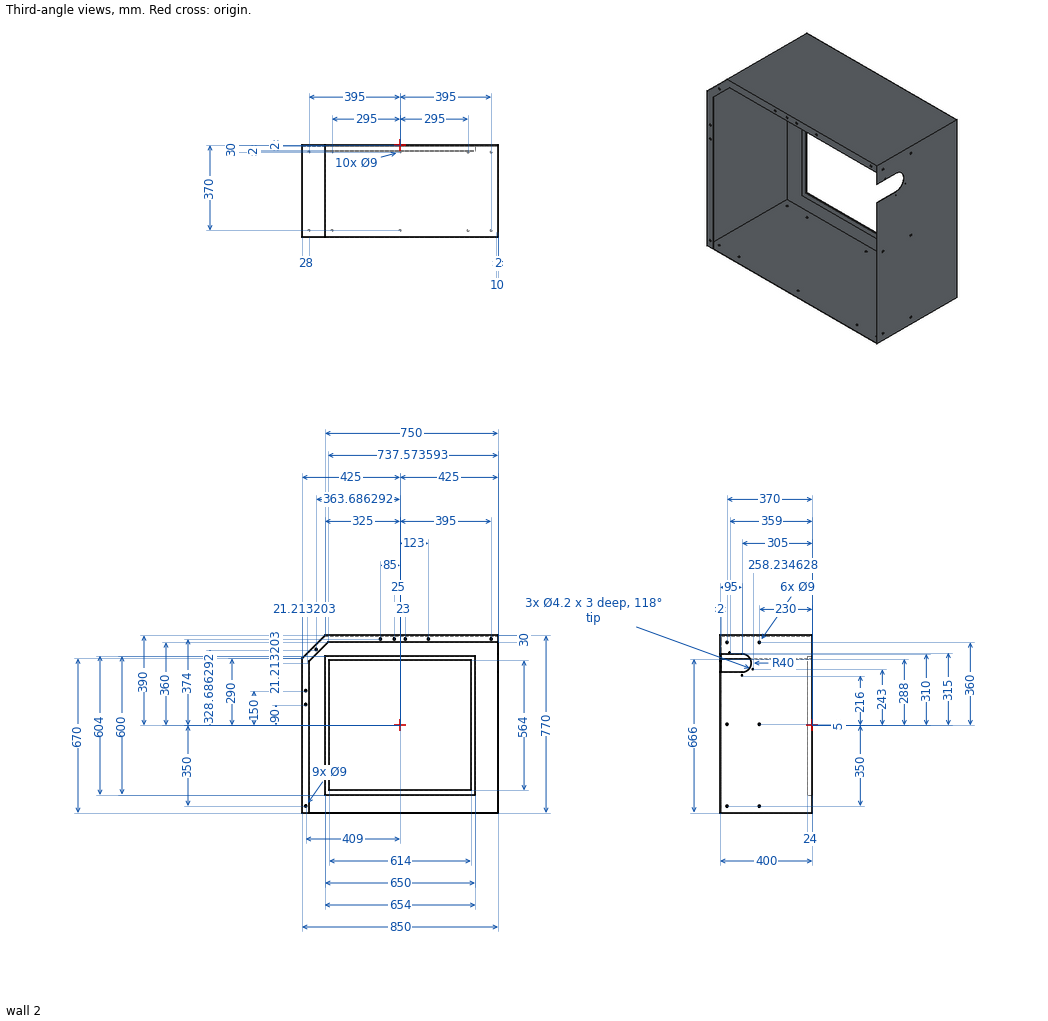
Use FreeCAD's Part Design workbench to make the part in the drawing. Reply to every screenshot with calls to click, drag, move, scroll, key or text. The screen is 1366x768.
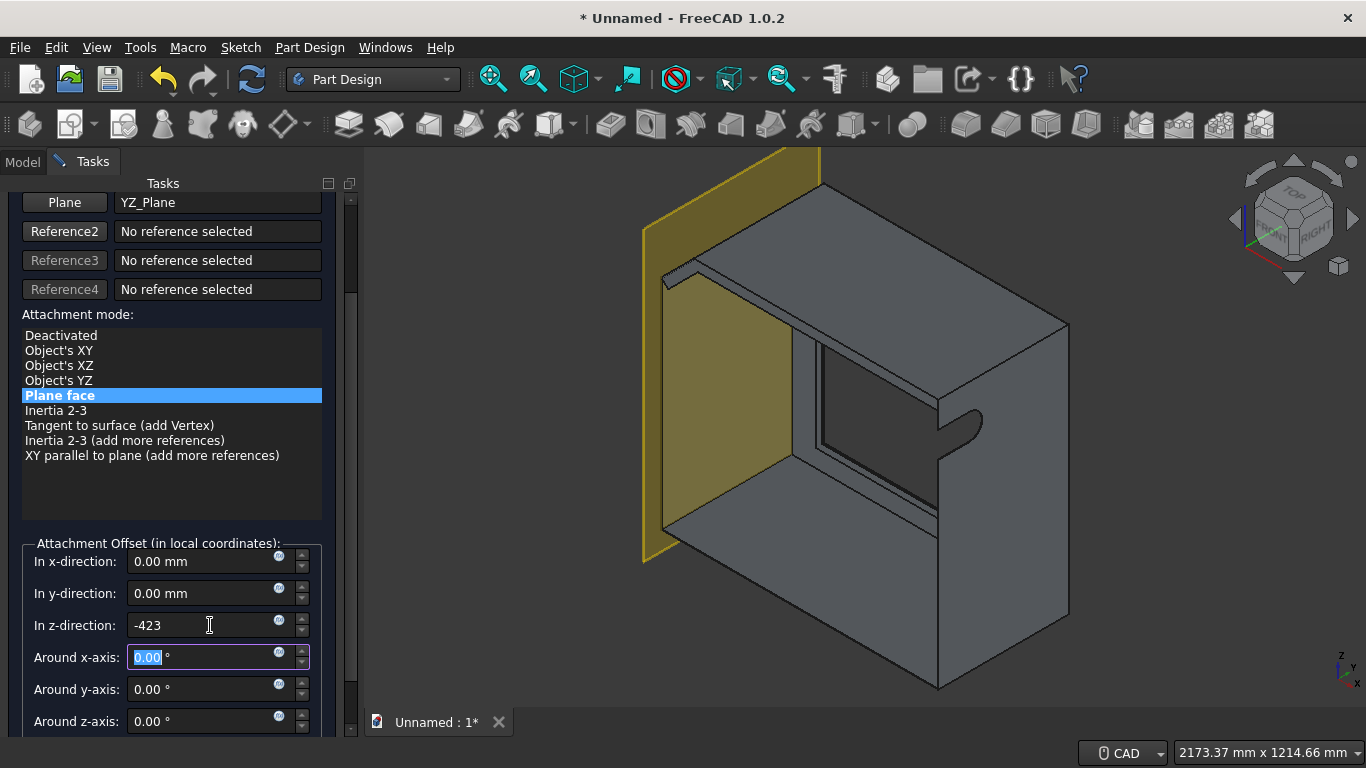
scroll(351, 464, up, 3)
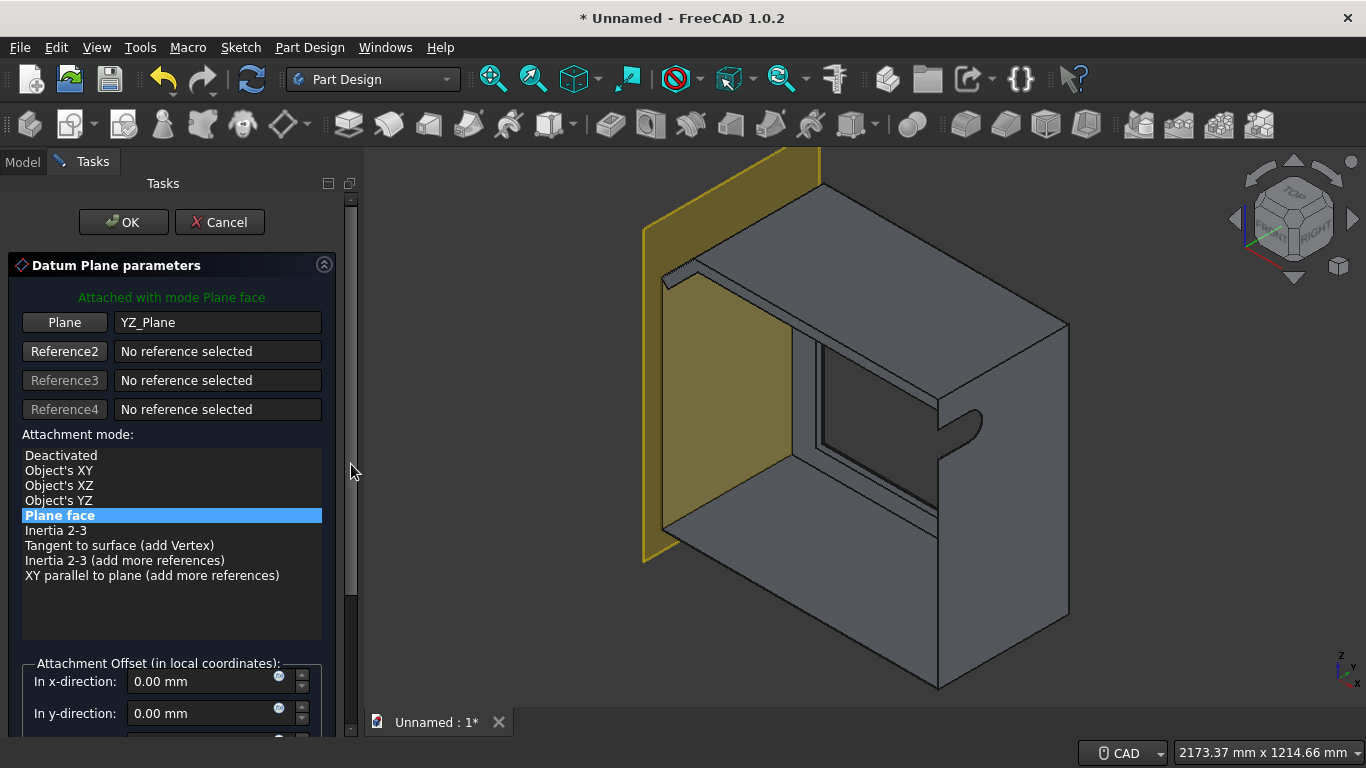
click(124, 222)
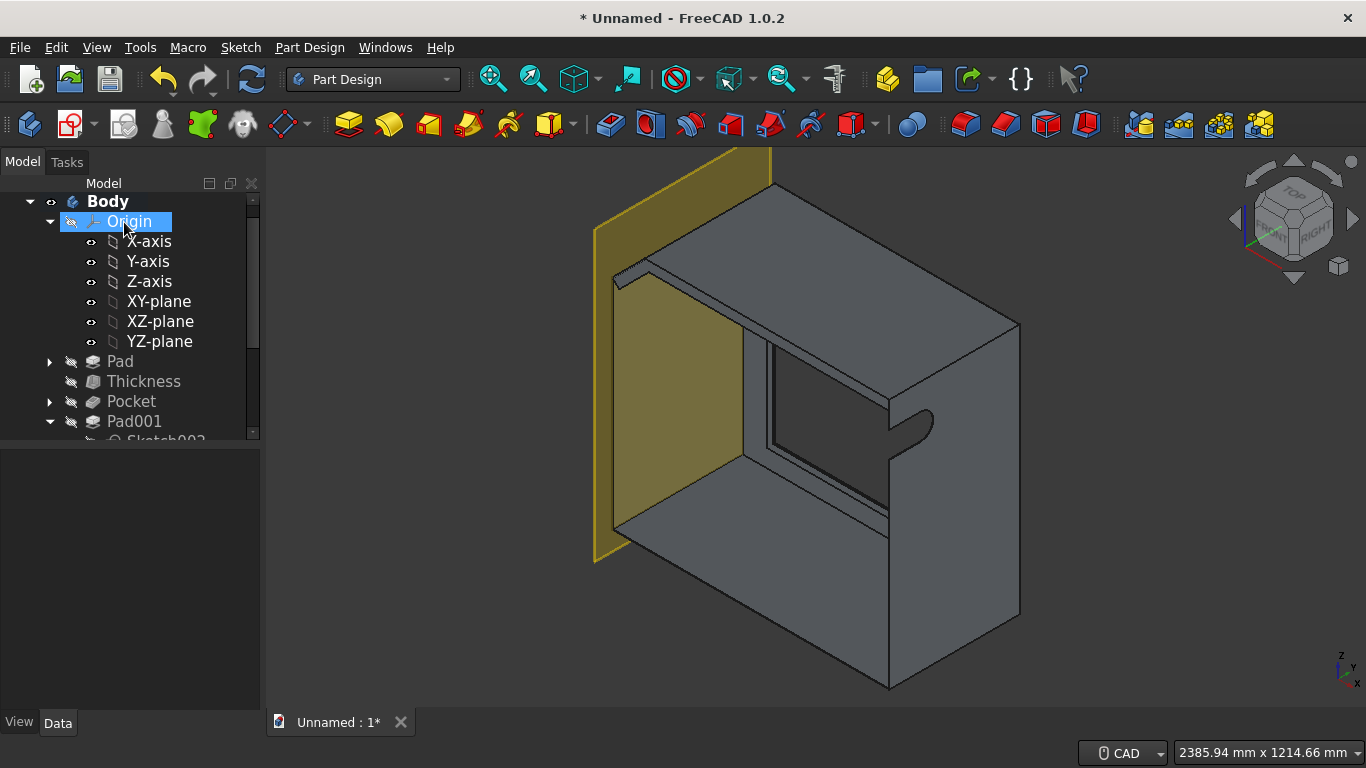
scroll(120, 317, down, 3)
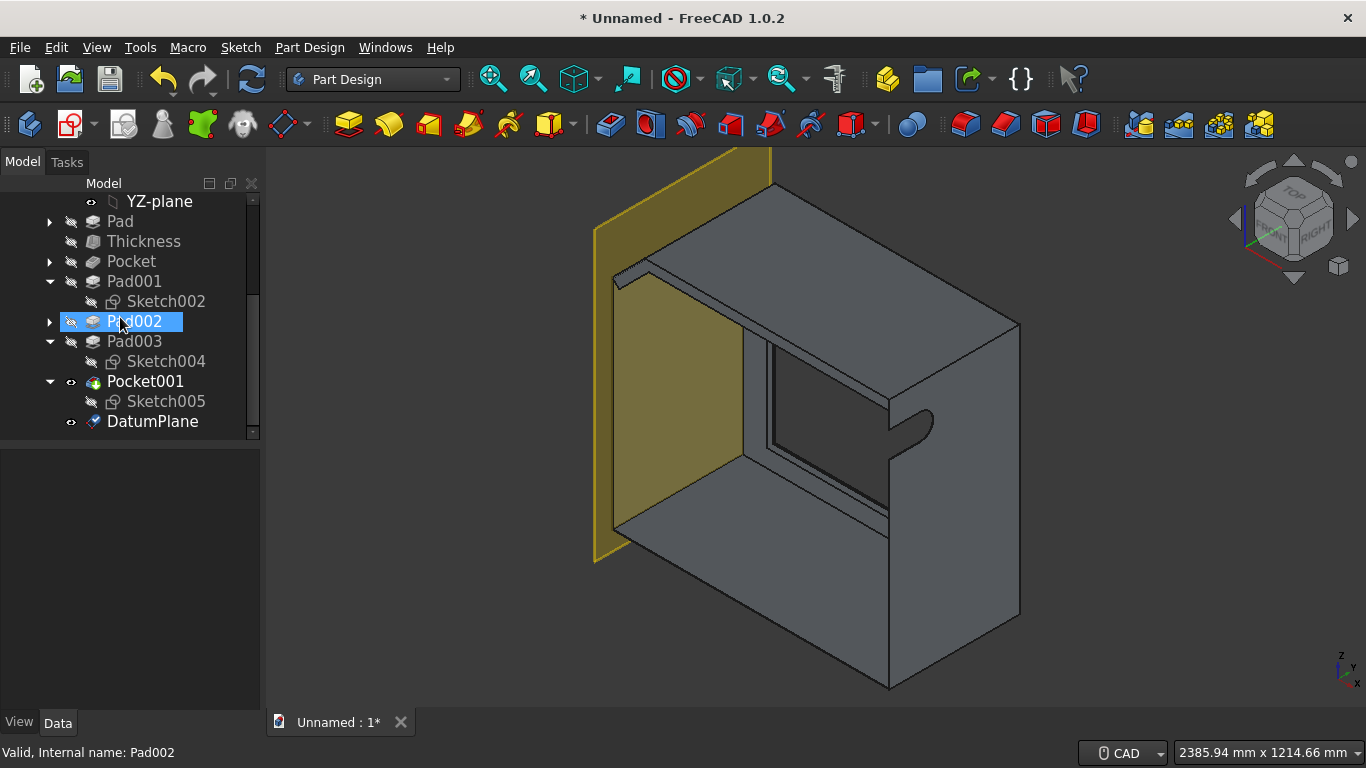
click(116, 422)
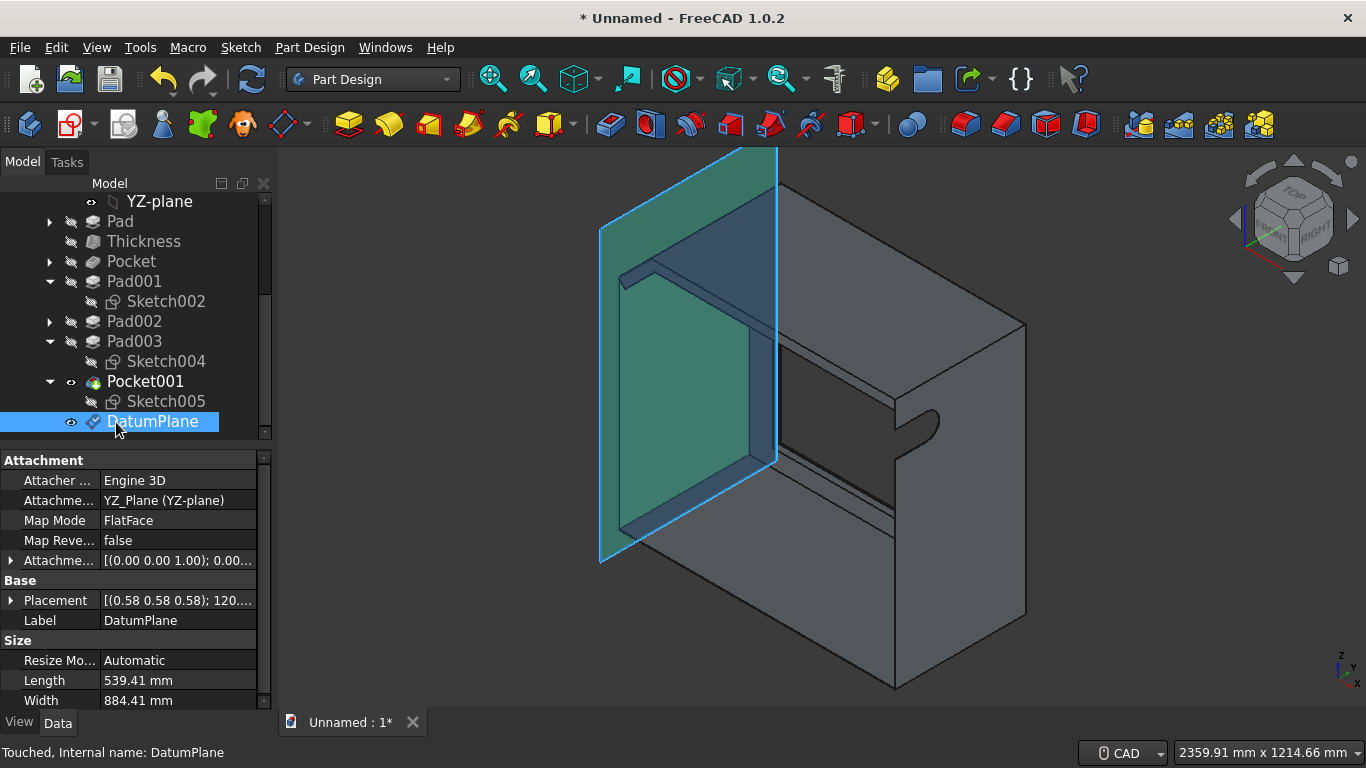
click(70, 124)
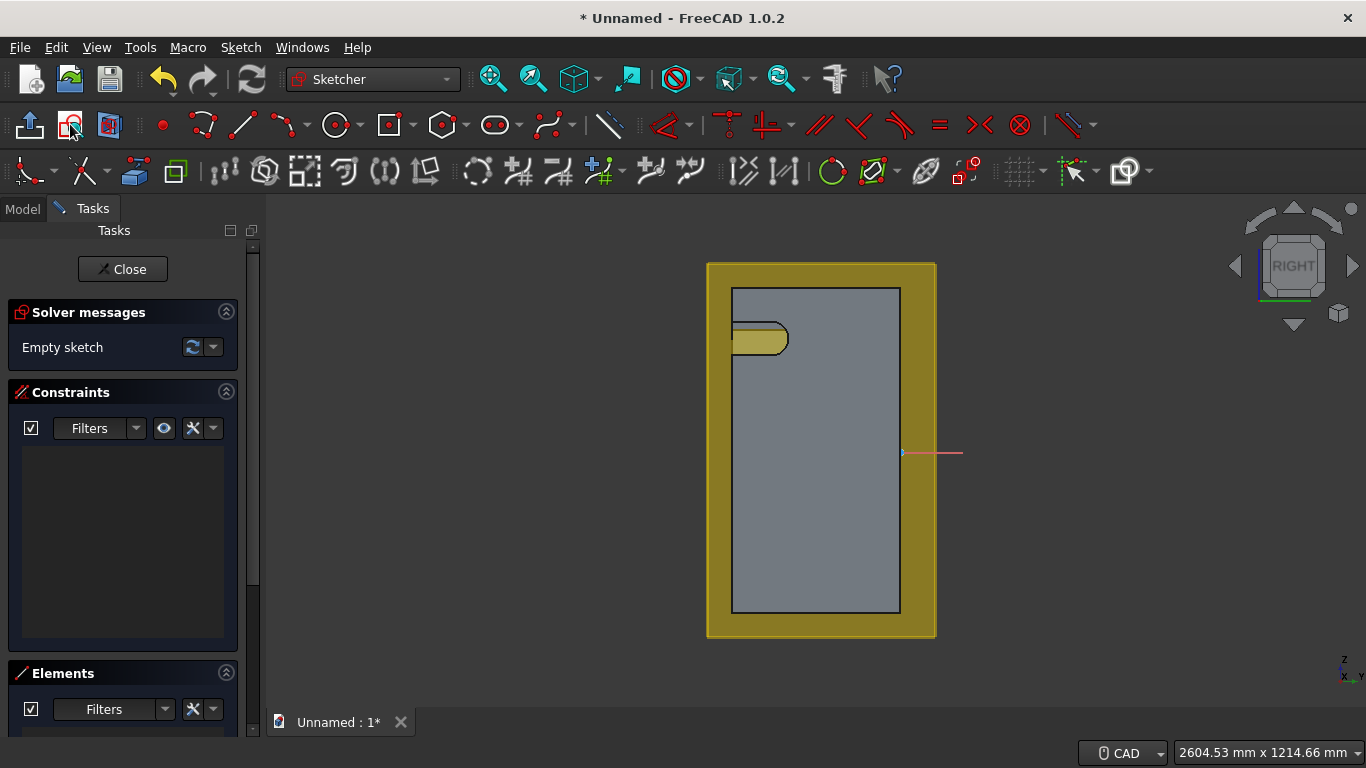
click(110, 126)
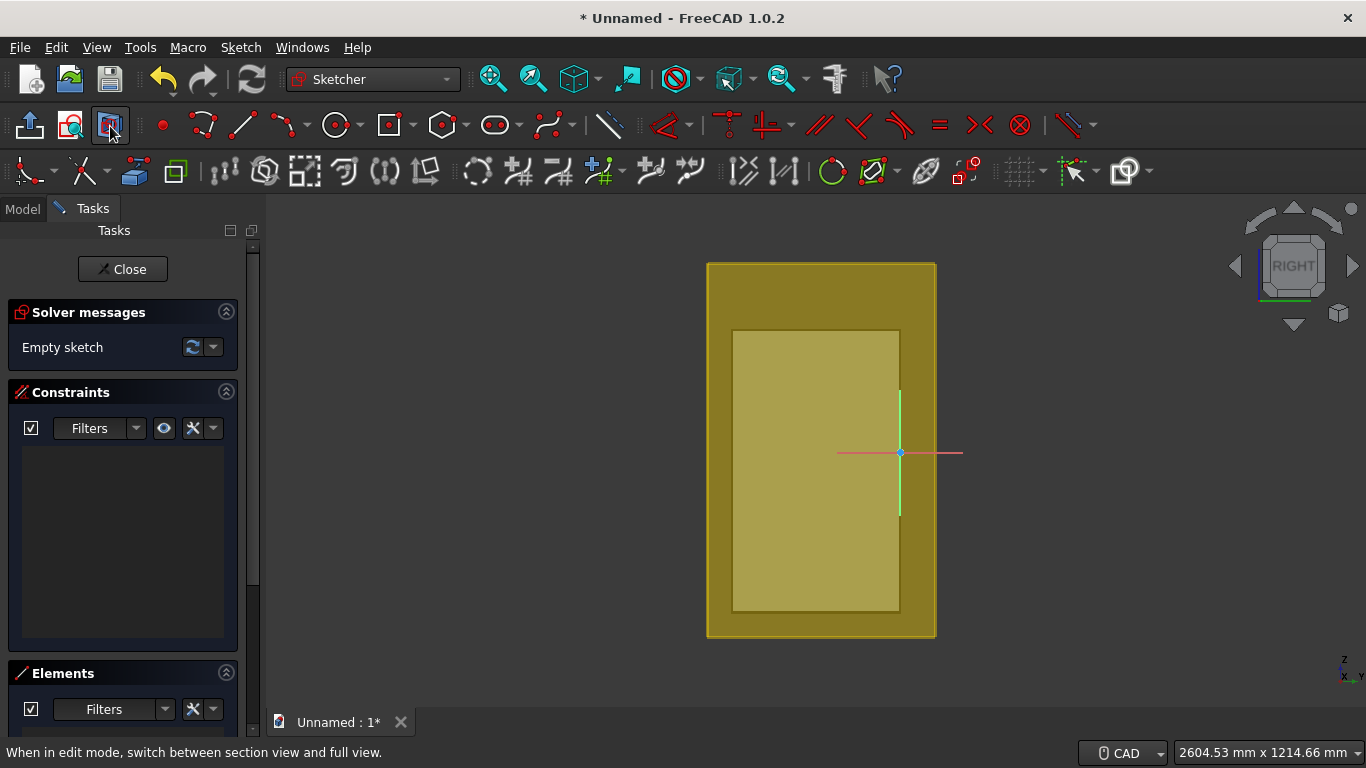
key(g)
key(r)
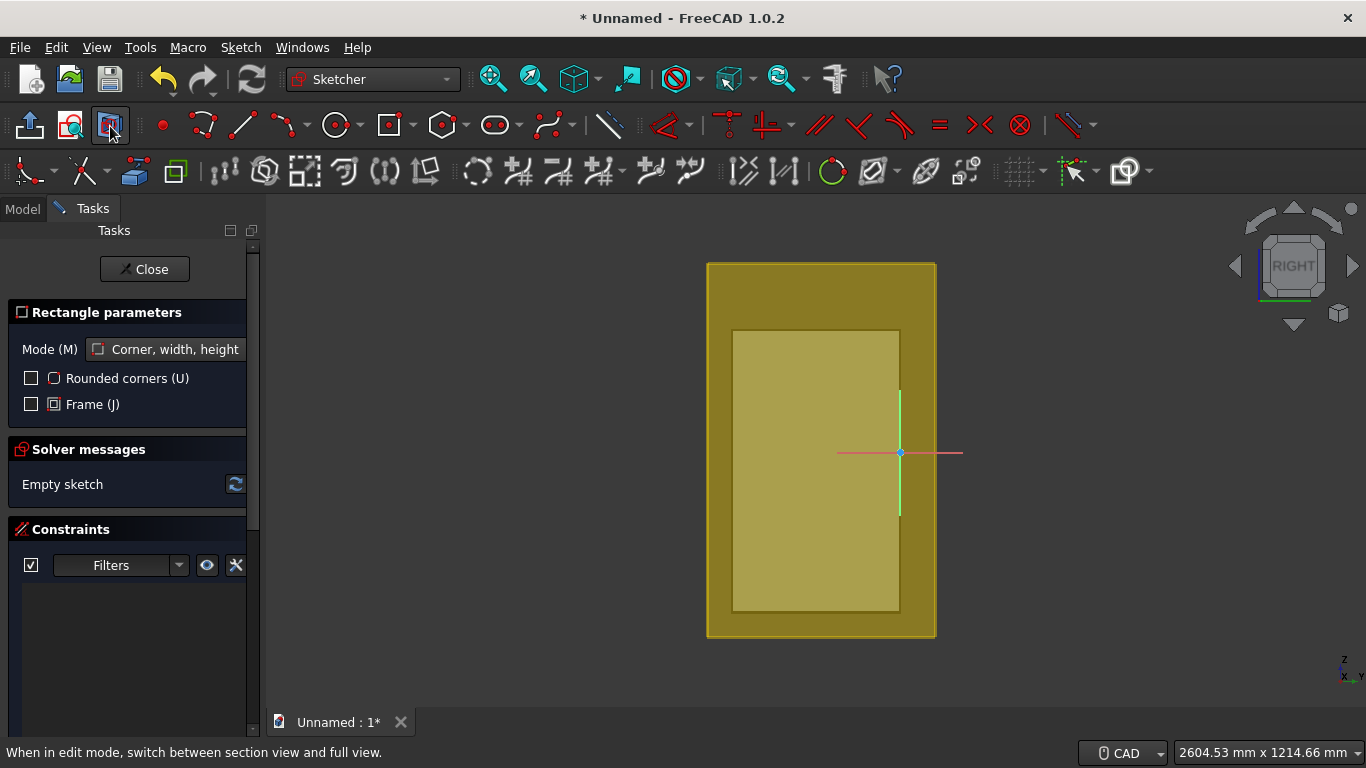
scroll(732, 331, up, 15)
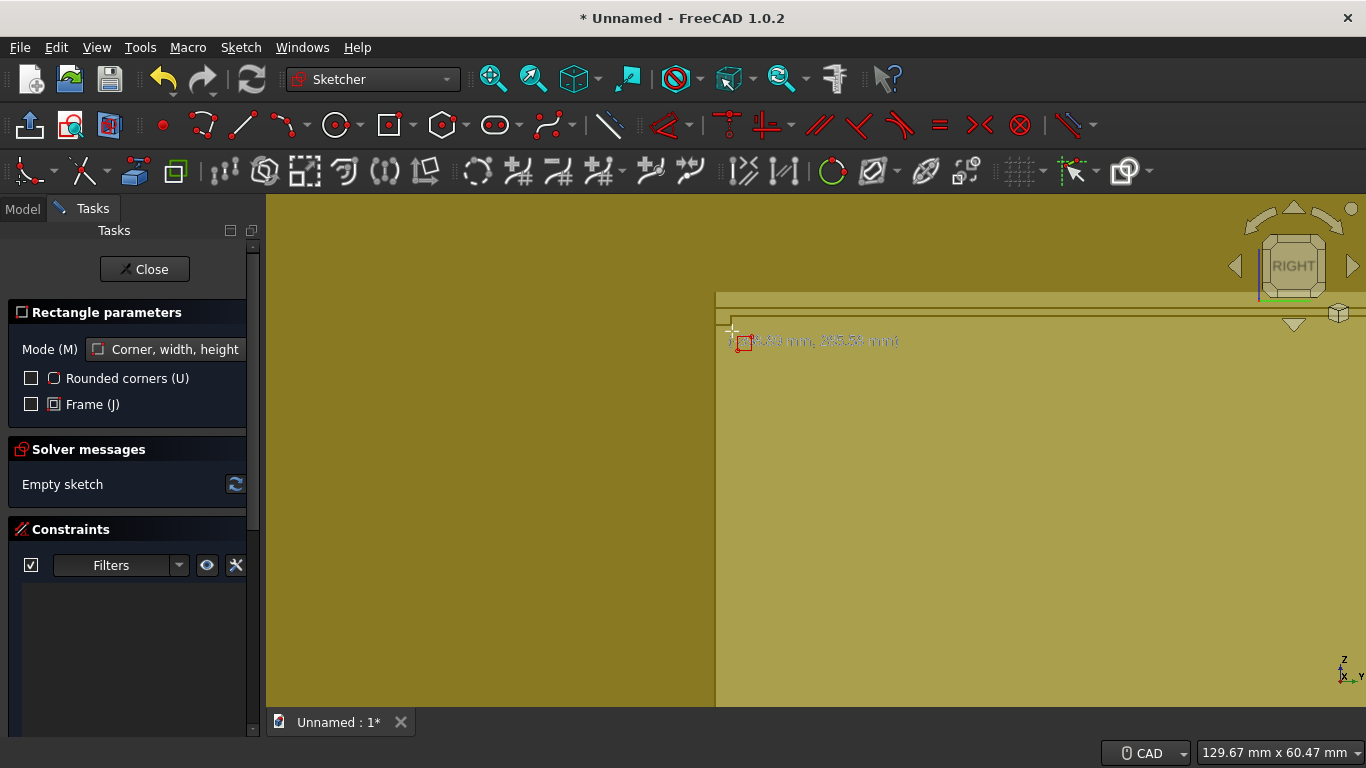
scroll(640, 276, down, 14)